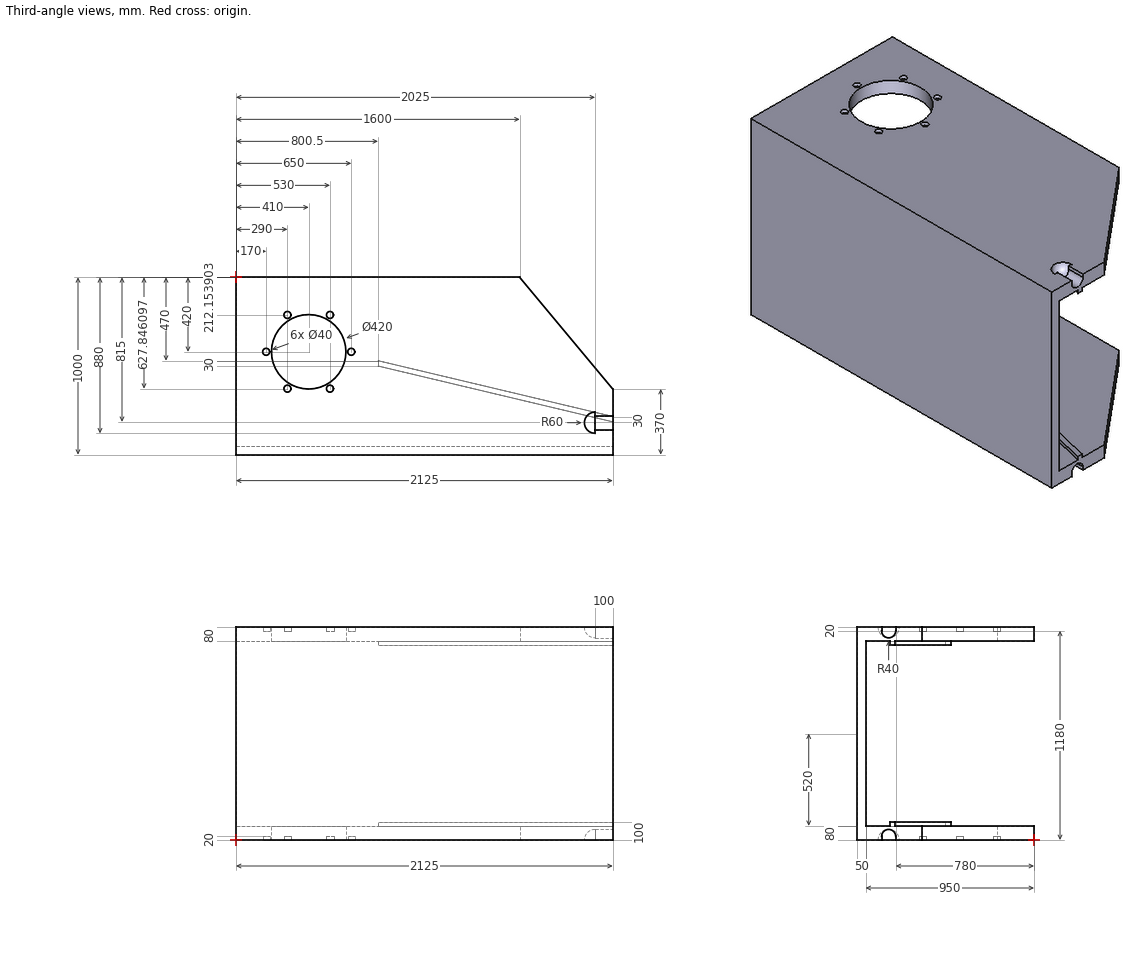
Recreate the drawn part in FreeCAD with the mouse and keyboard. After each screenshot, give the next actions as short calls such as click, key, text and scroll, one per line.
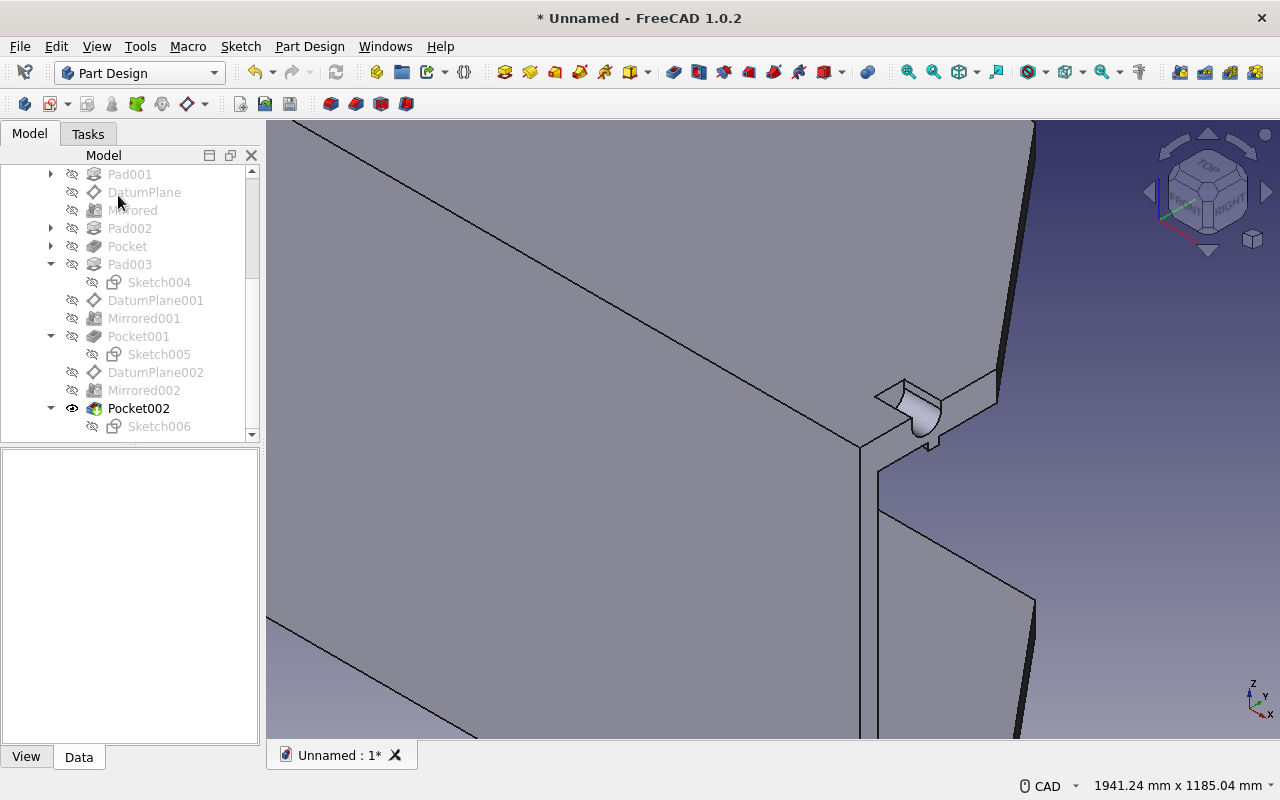
key(v)
key(f)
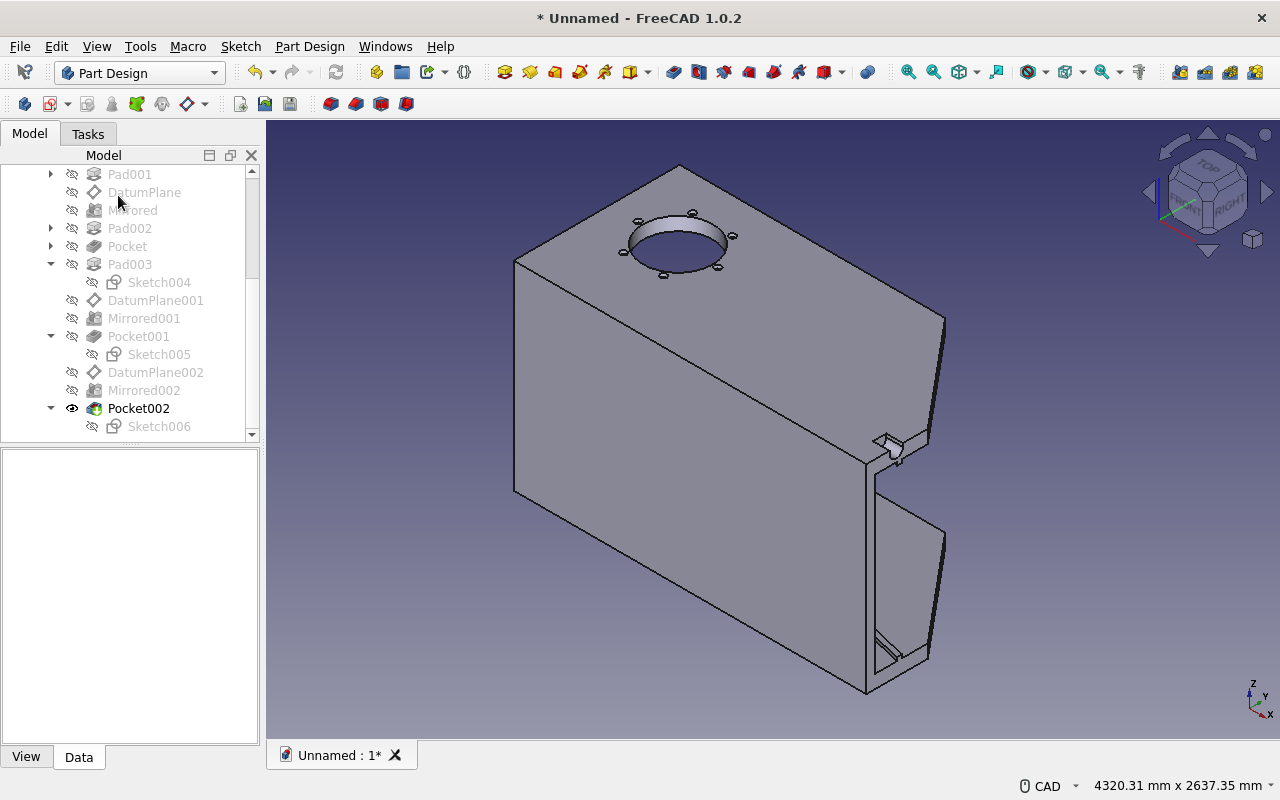
click(823, 343)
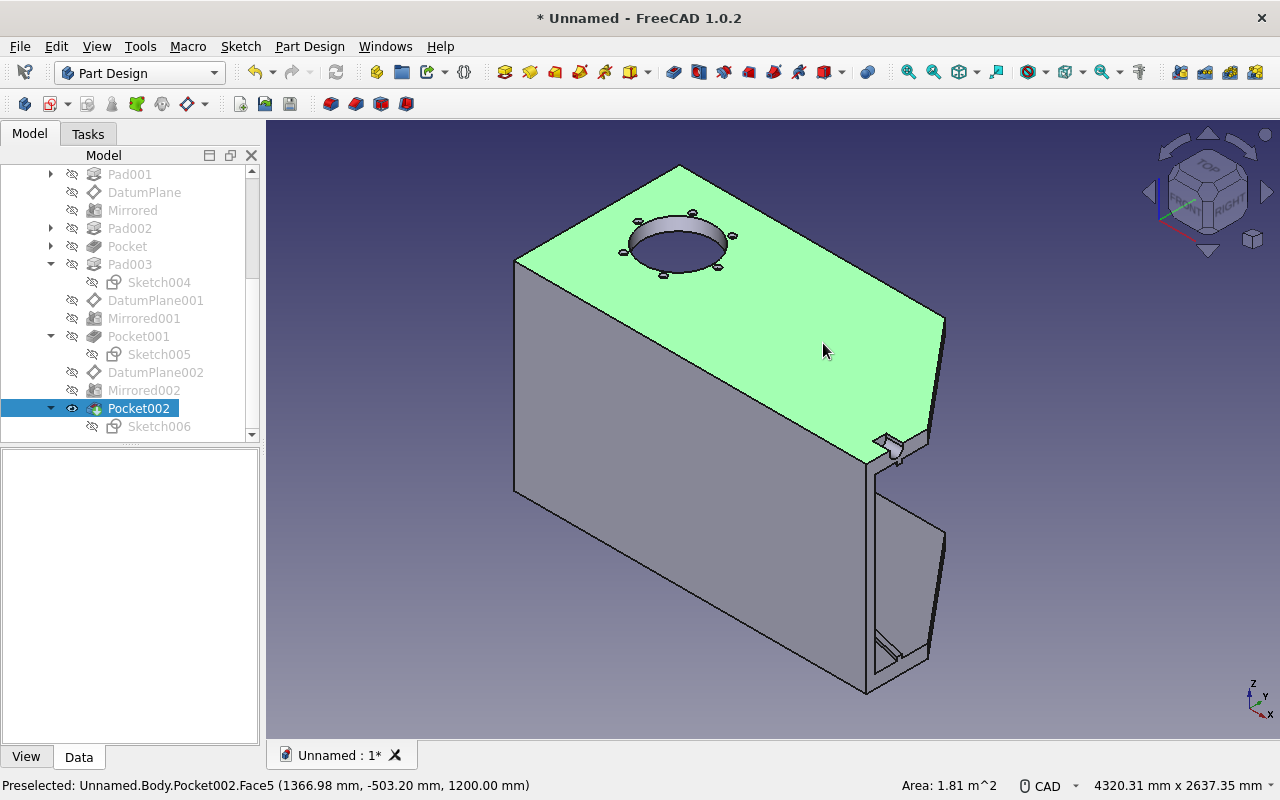
click(50, 104)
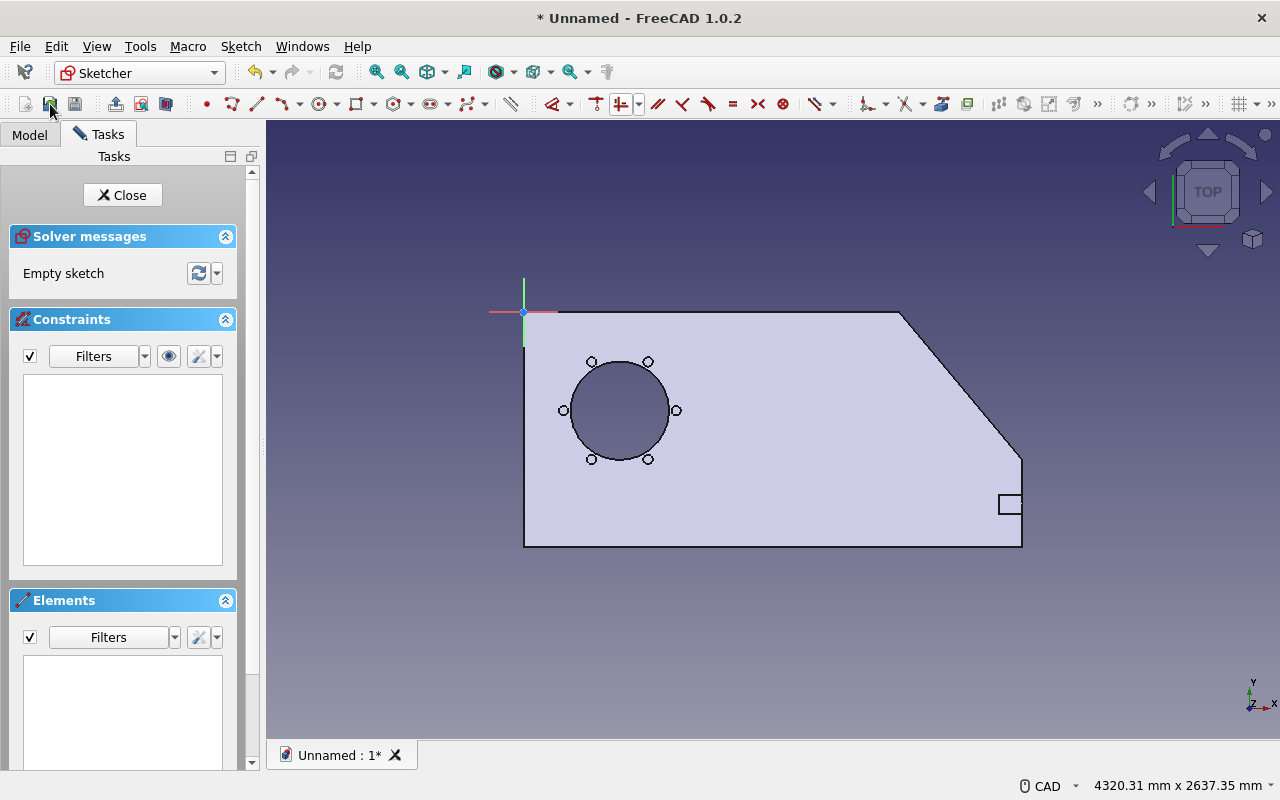
scroll(1021, 518, up, 12)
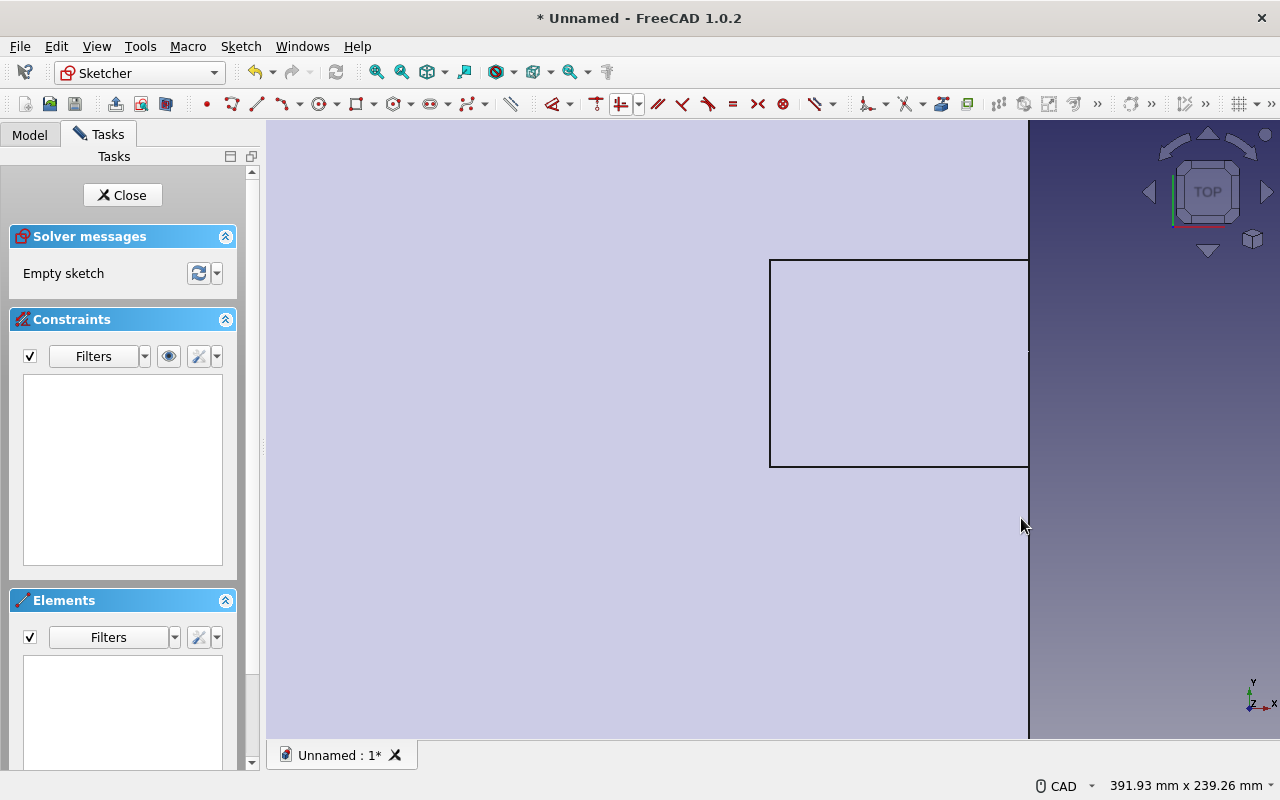
key(g)
key(l)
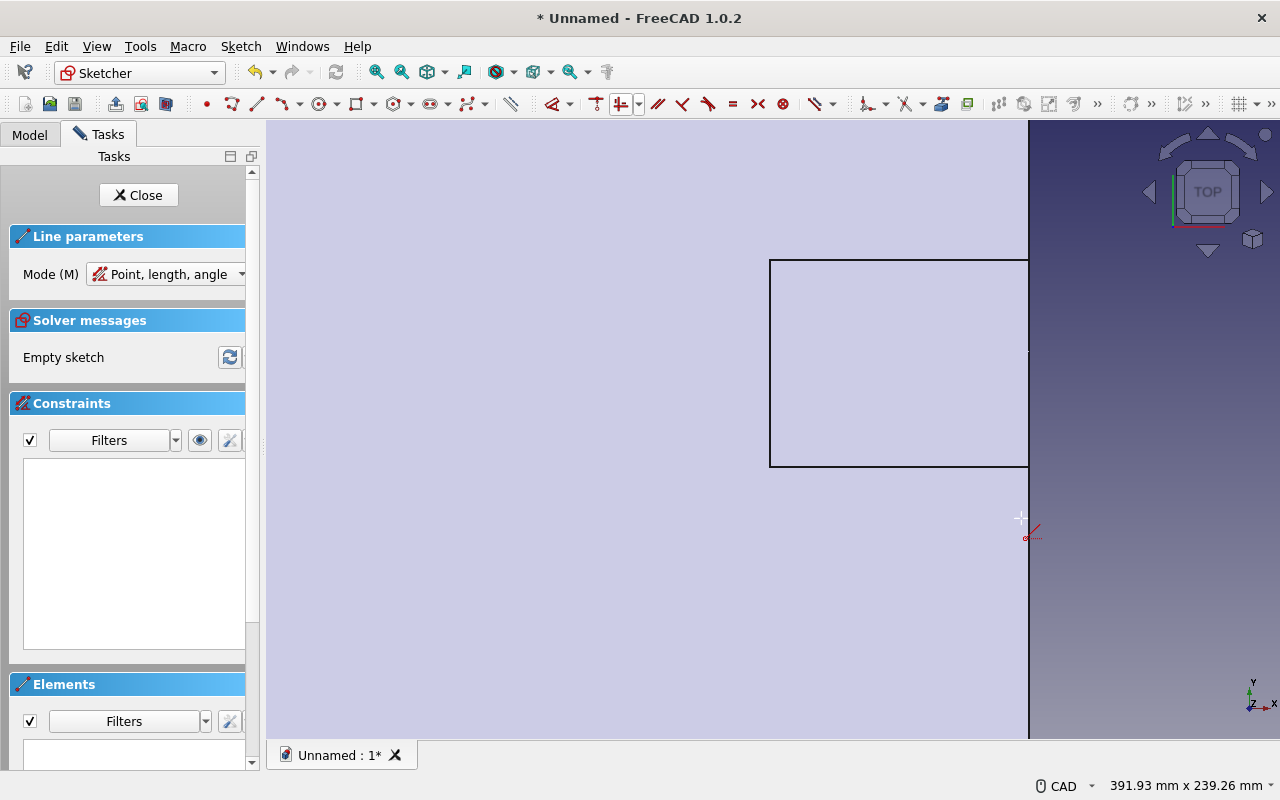
click(770, 519)
click(770, 209)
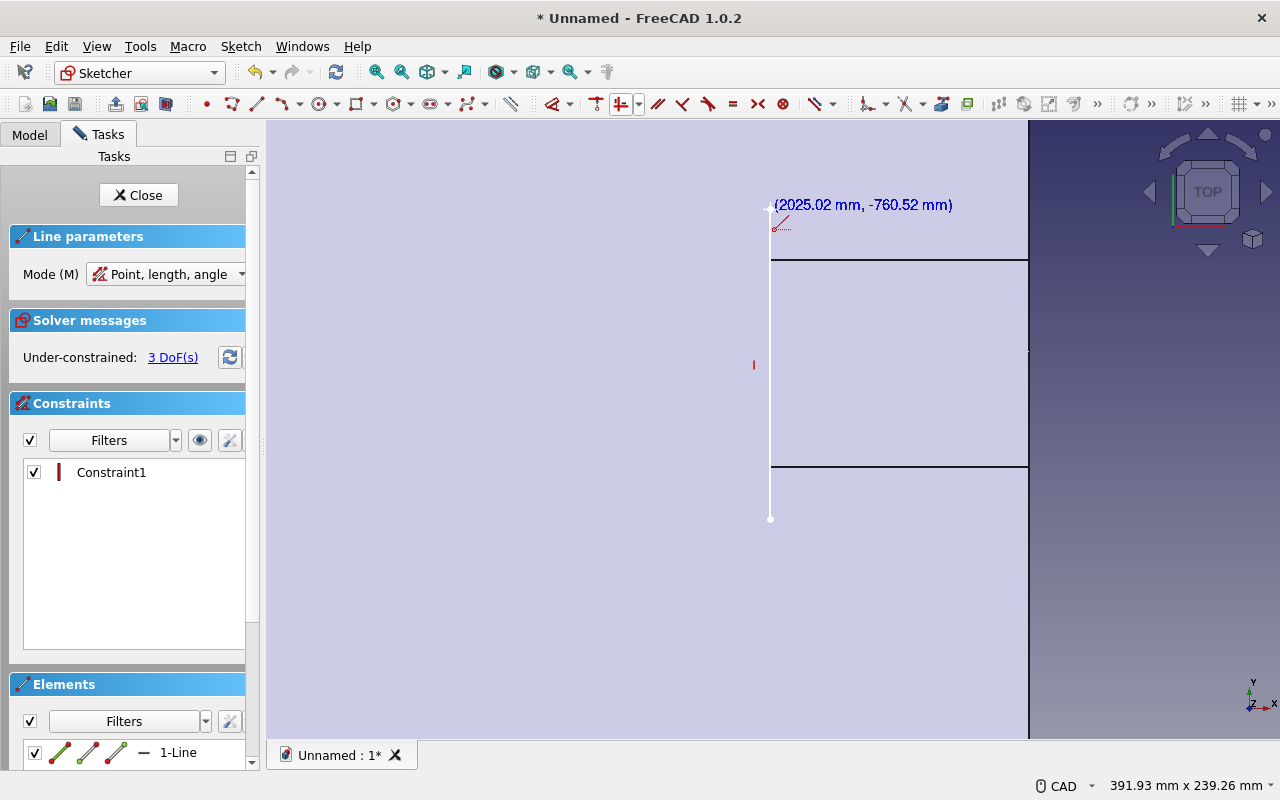
click(282, 104)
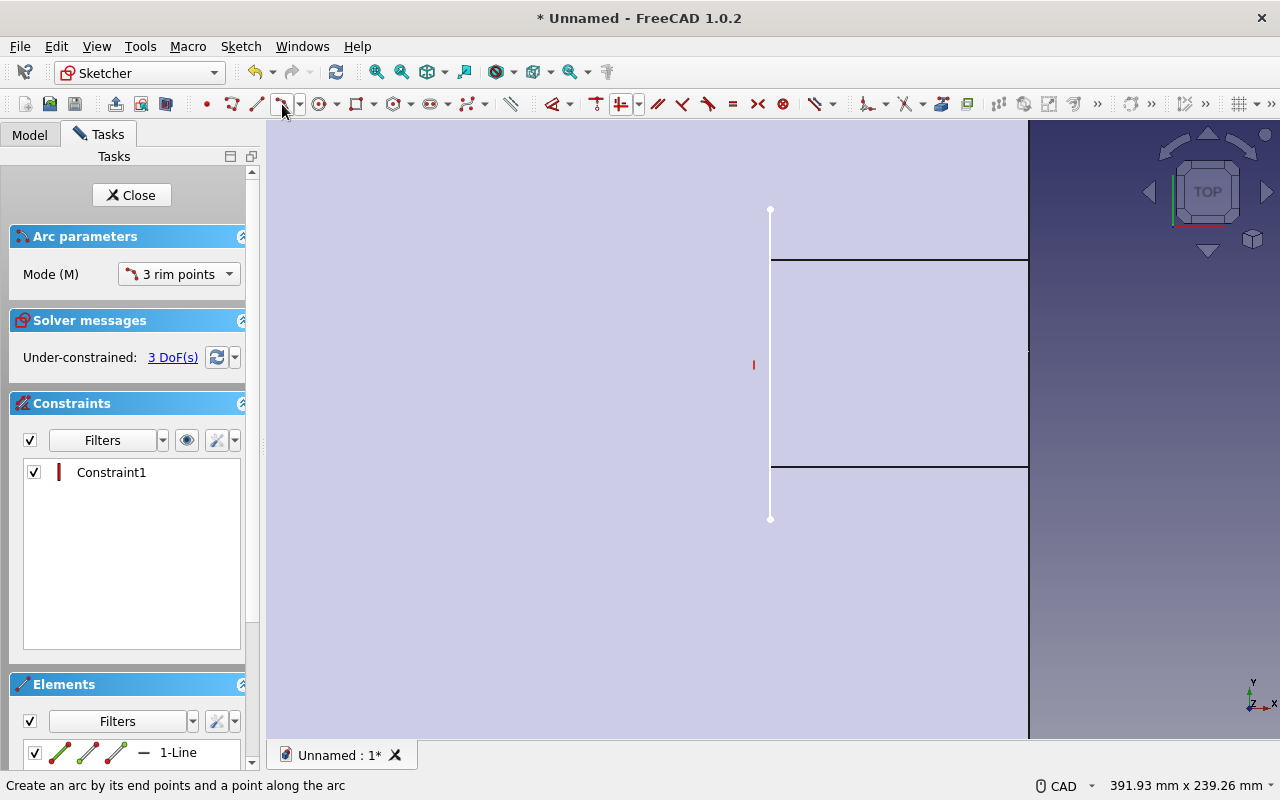
click(770, 210)
click(770, 520)
click(615, 364)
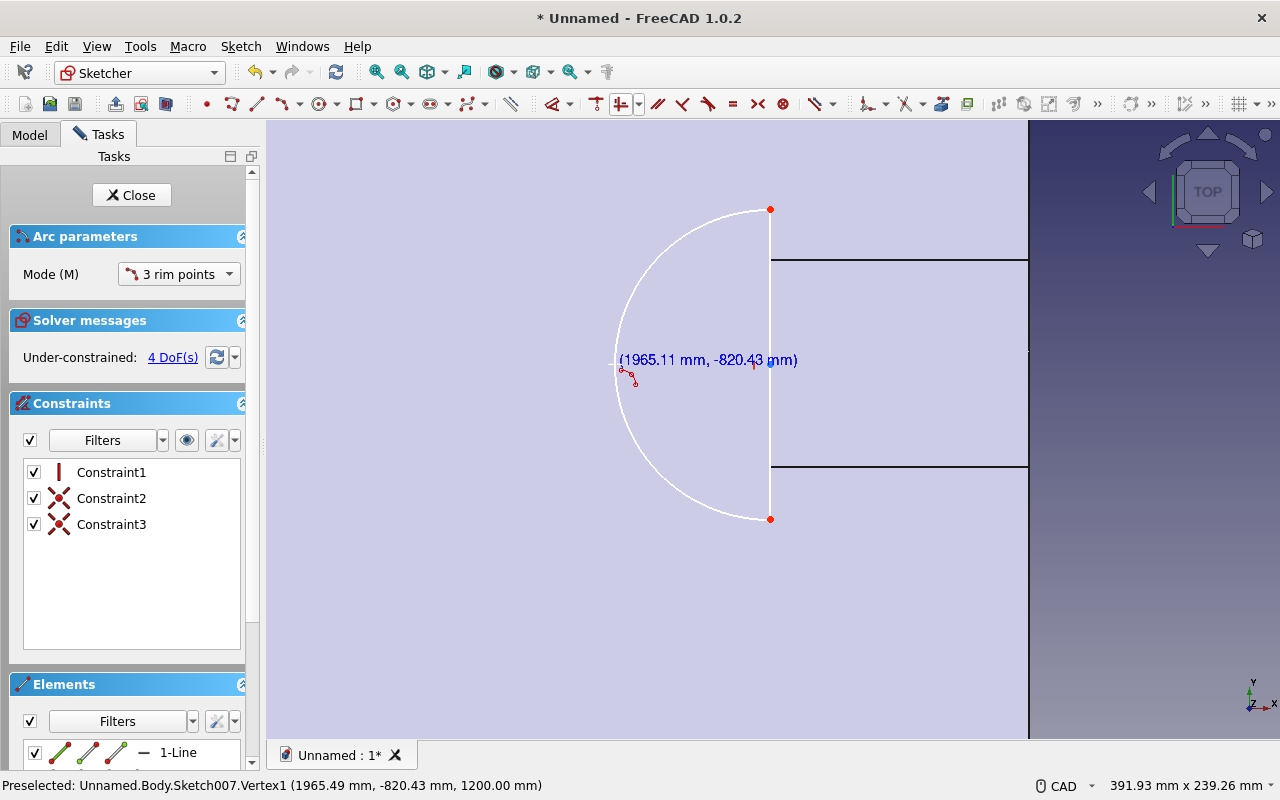
key(g)
key(l)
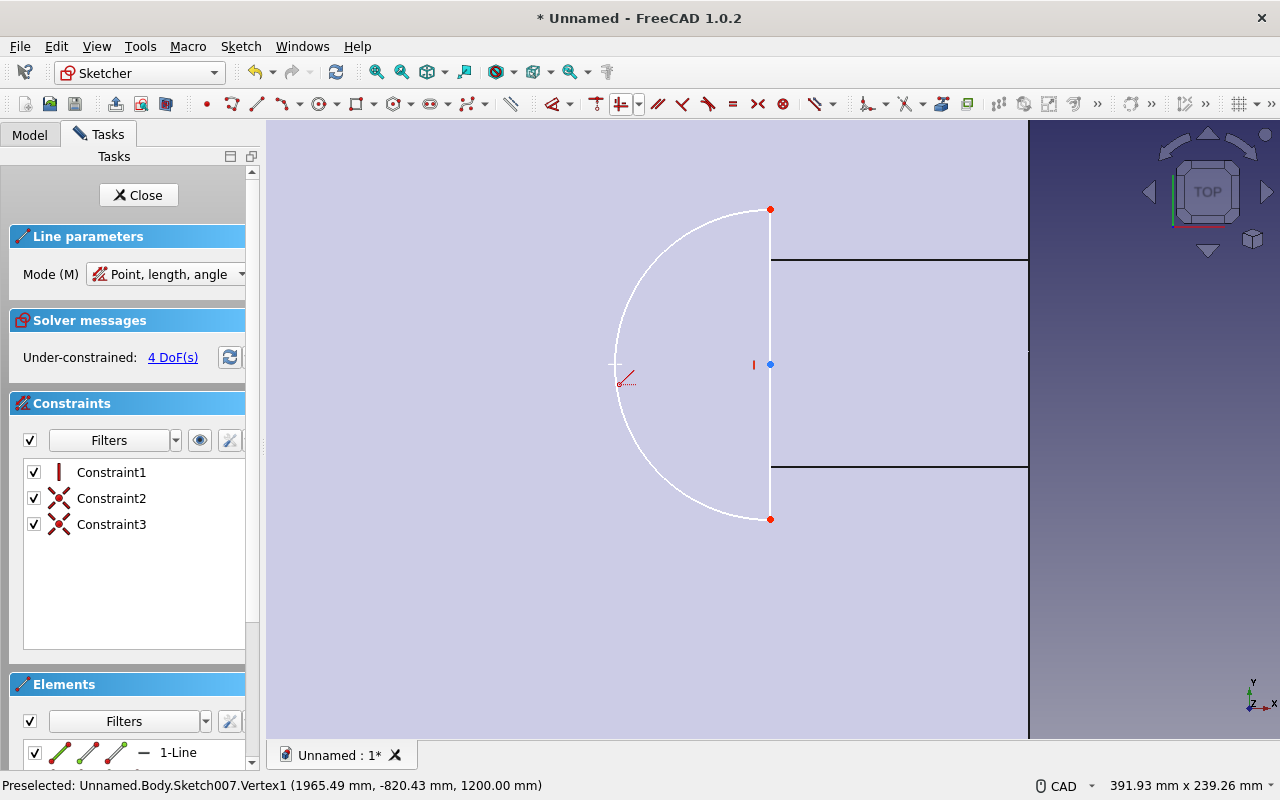
click(770, 550)
click(770, 643)
key(Escape)